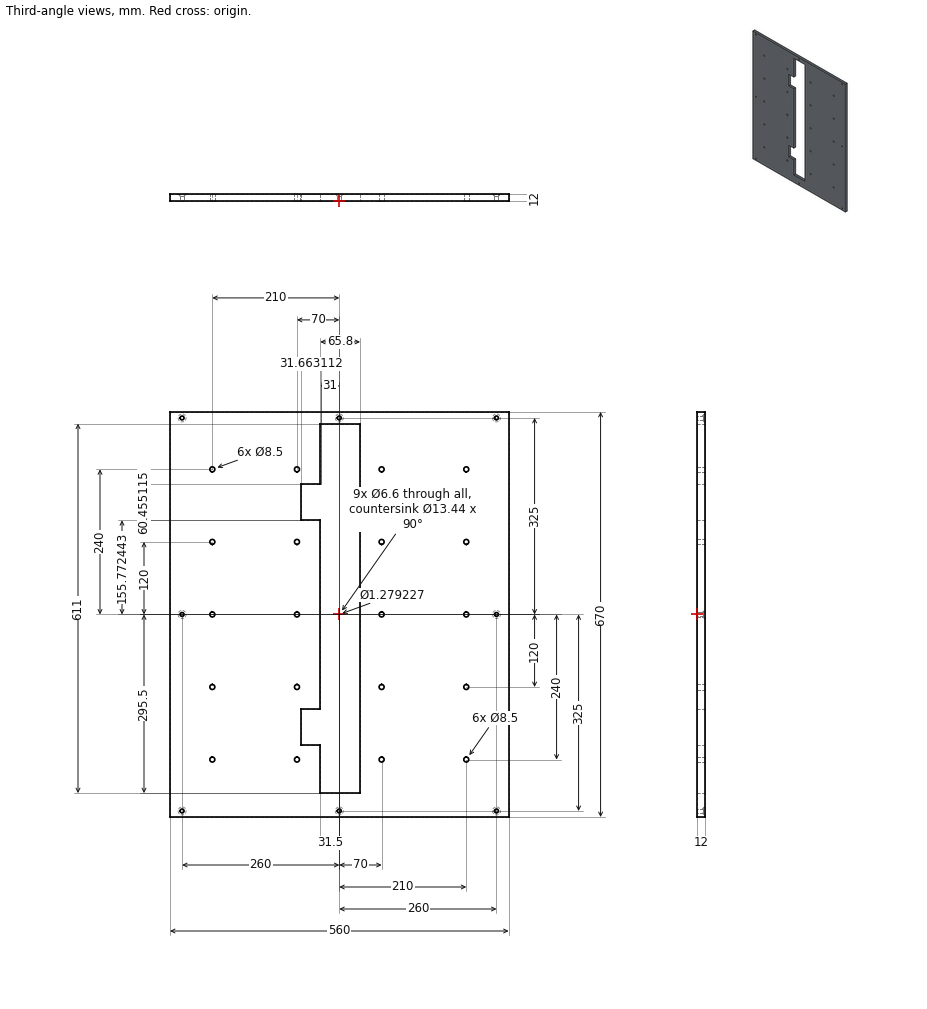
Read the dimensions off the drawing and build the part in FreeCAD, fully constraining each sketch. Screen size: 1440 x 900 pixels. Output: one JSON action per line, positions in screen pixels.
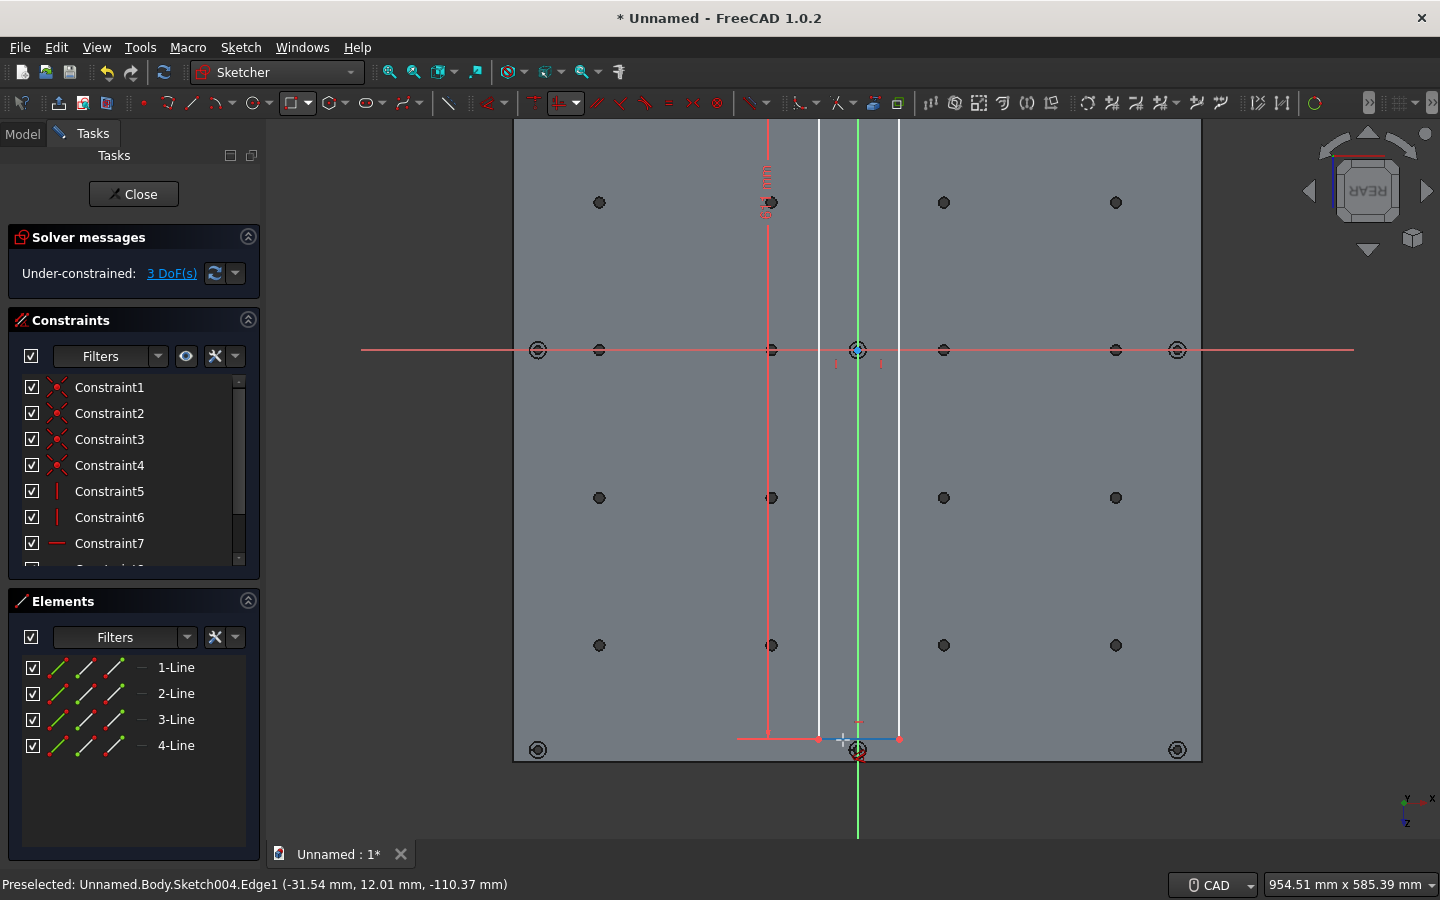
{"action": "left_click", "coordinate": [843, 739]}
{"action": "left_click", "coordinate": [841, 773]}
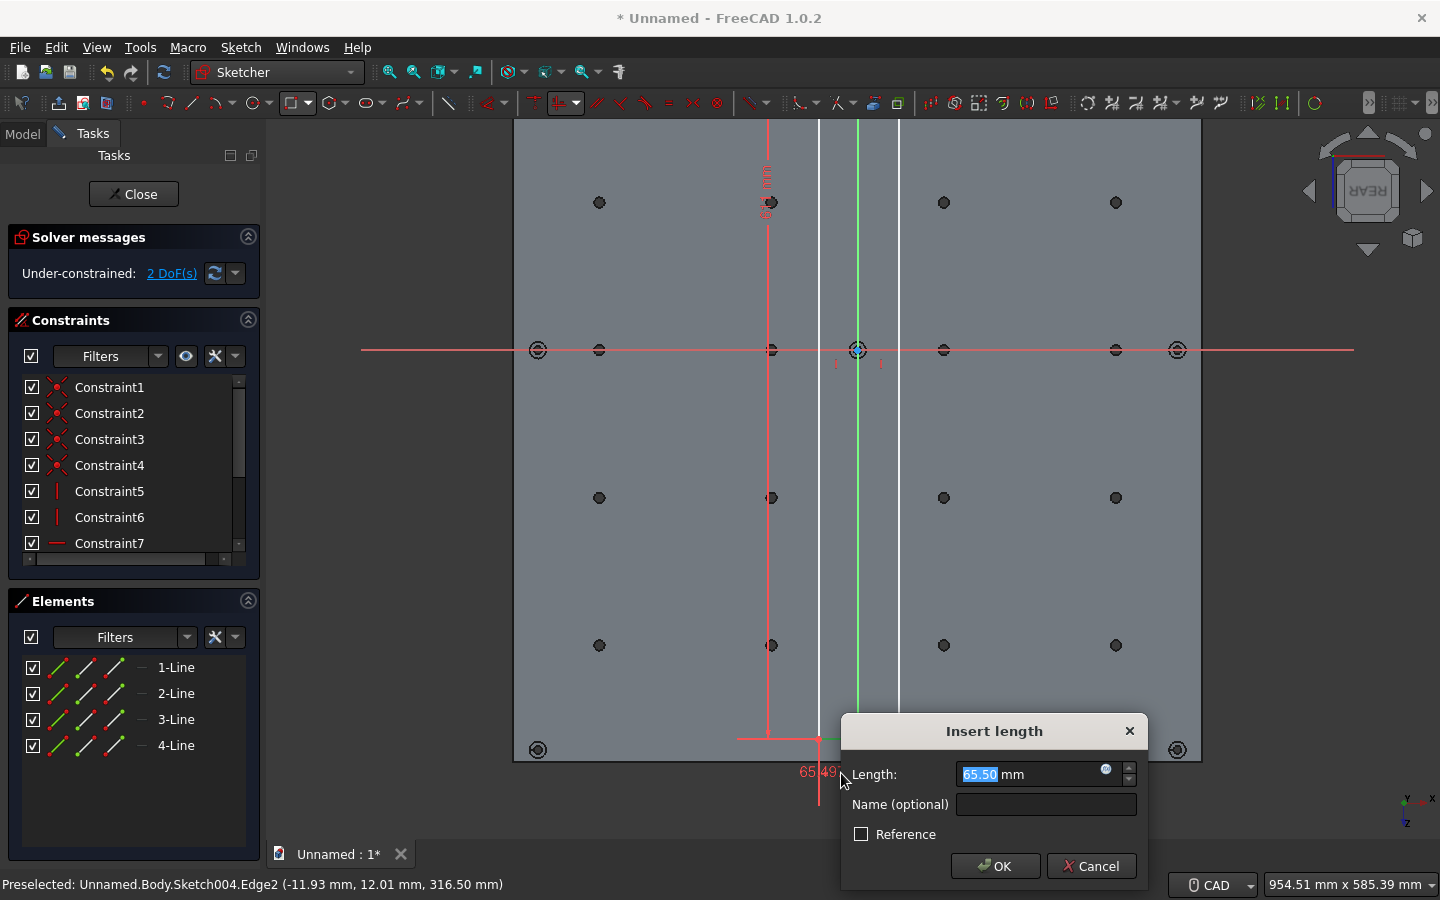
{"action": "type", "text": "65.8"}
{"action": "key", "text": "Return"}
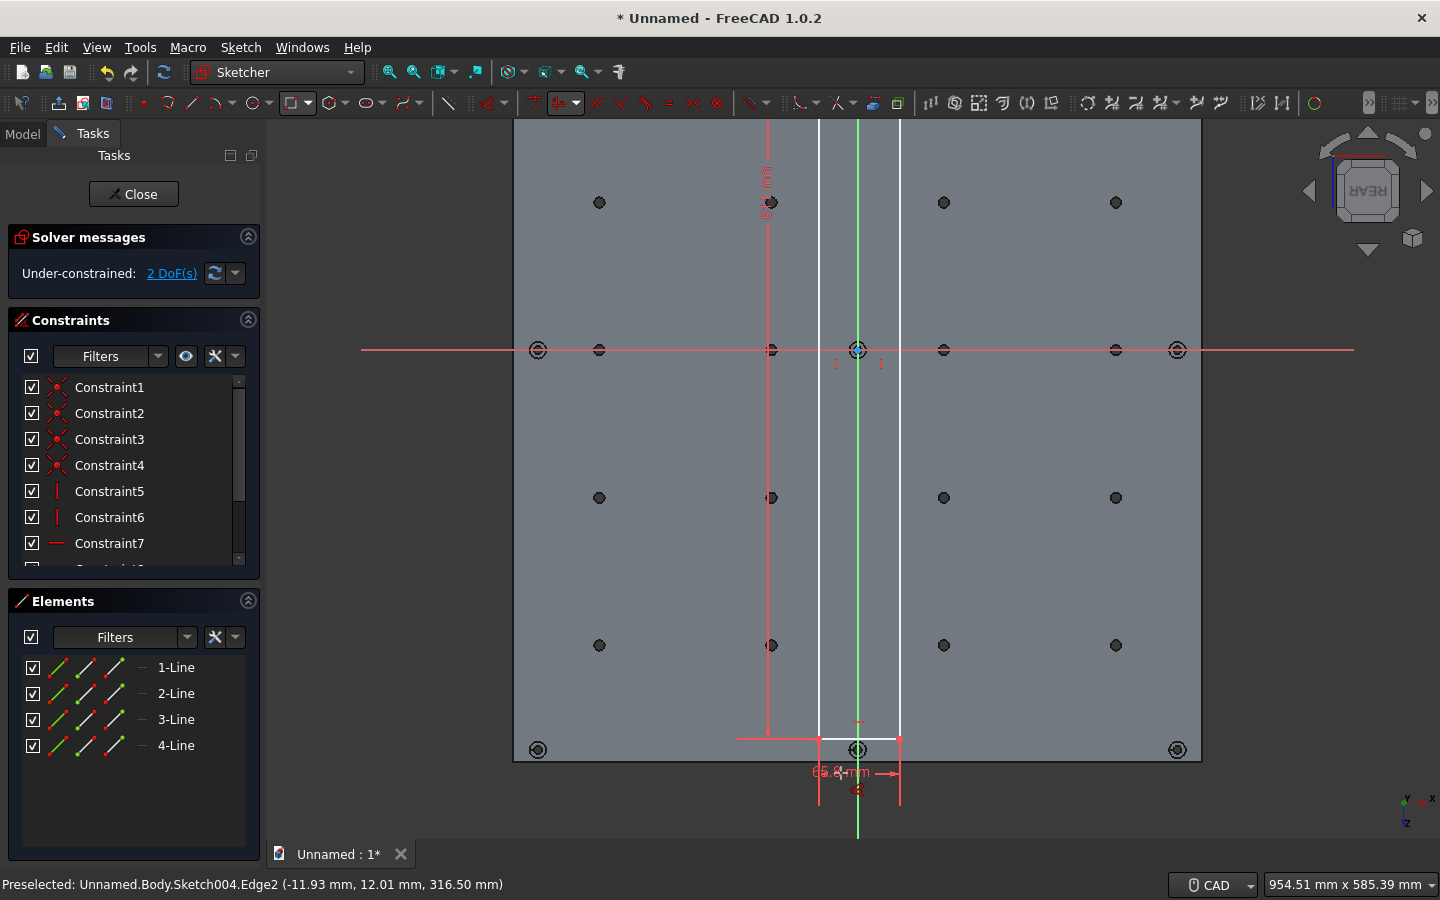
{"action": "scroll", "coordinate": [632, 716], "scroll_direction": "down", "scroll_amount": 2}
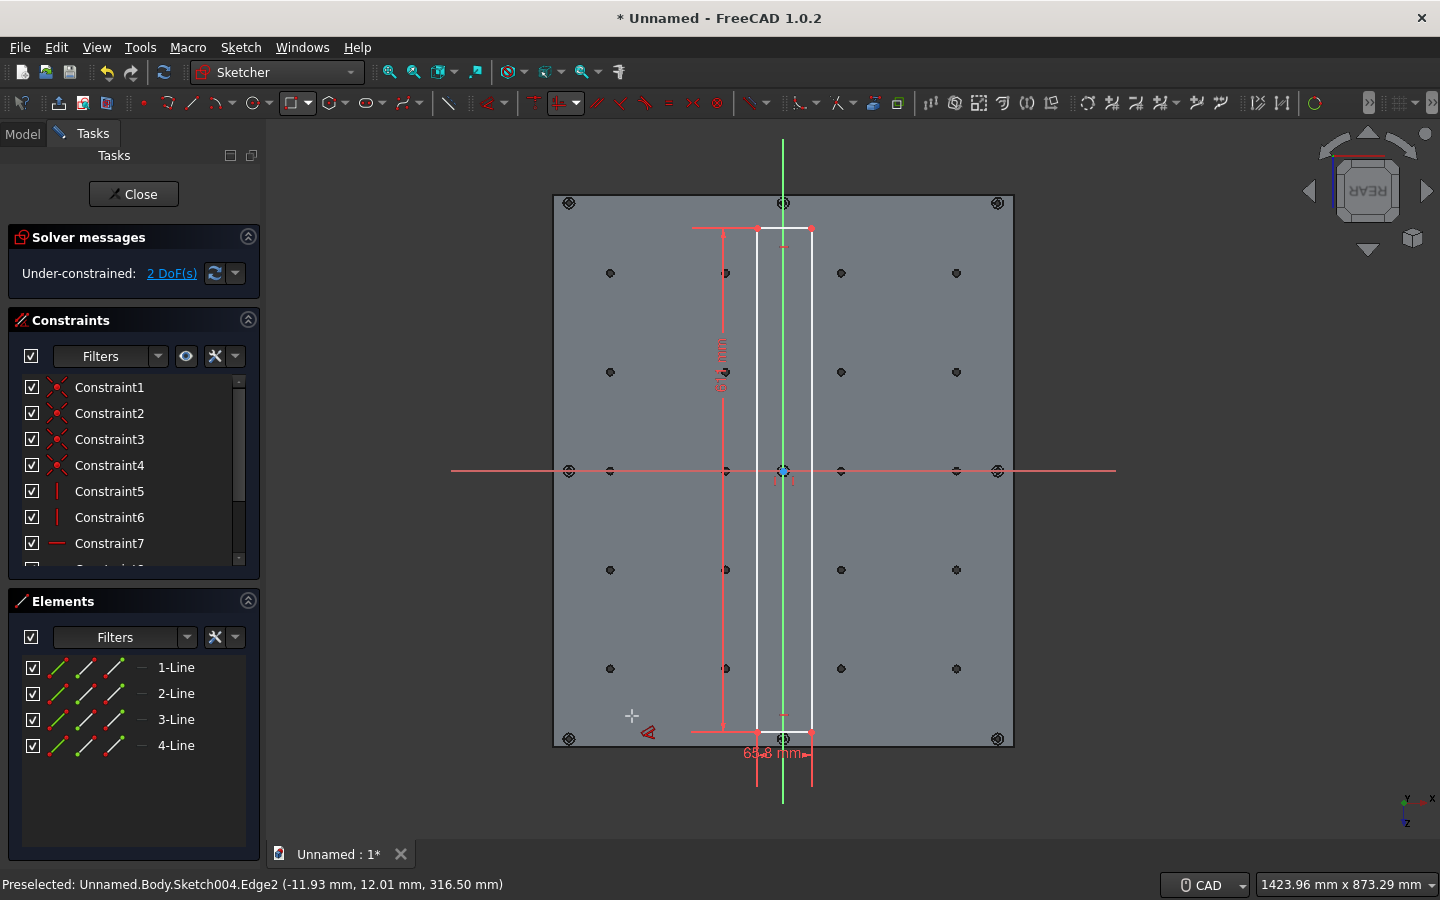
{"action": "scroll", "coordinate": [757, 228], "scroll_direction": "up", "scroll_amount": 3}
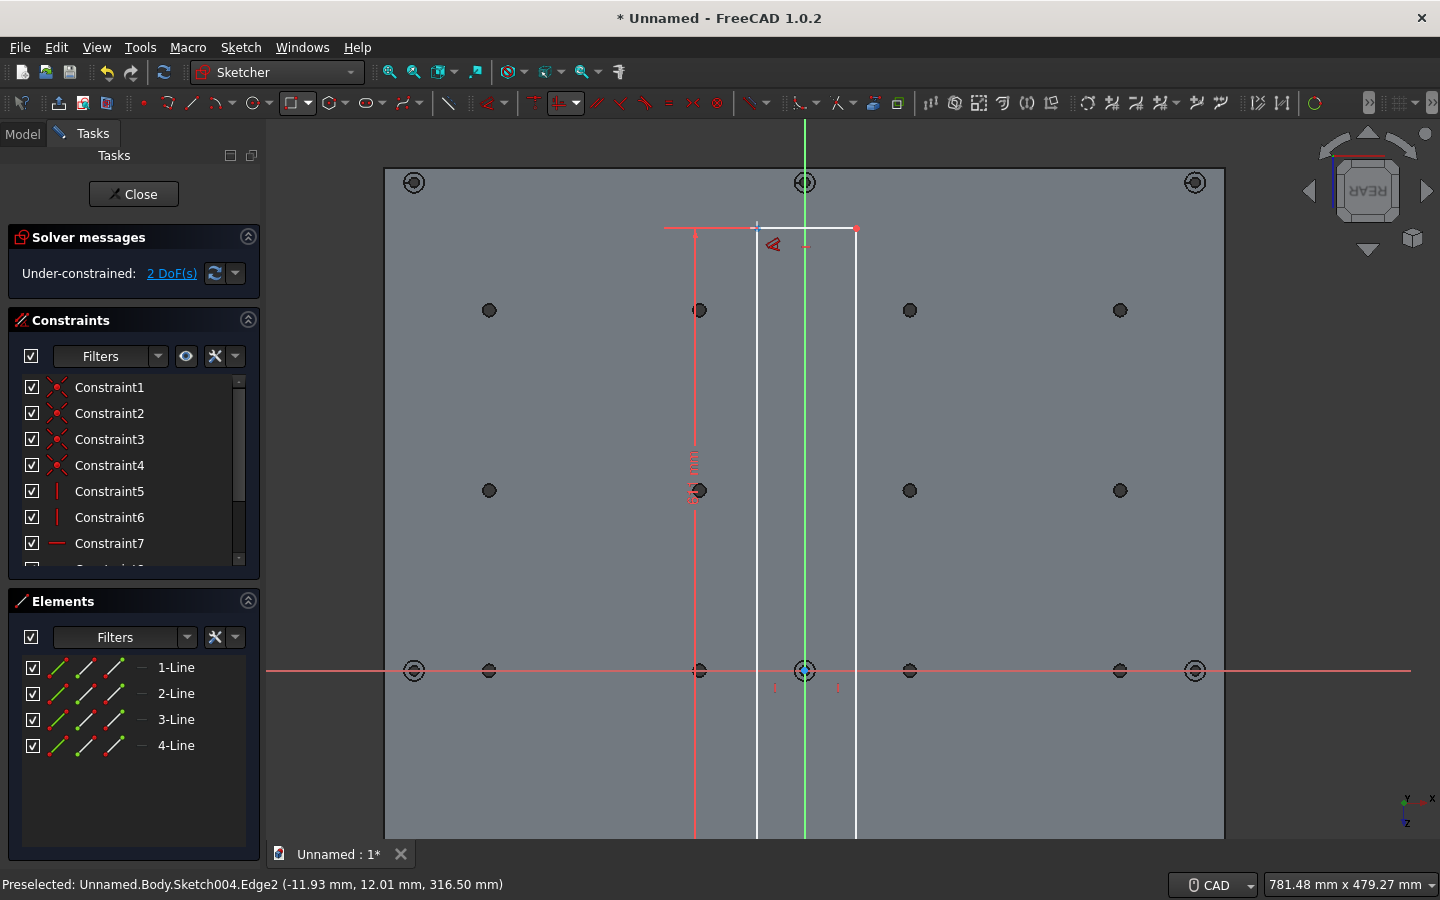
{"action": "left_click", "coordinate": [757, 228]}
{"action": "left_click", "coordinate": [781, 194]}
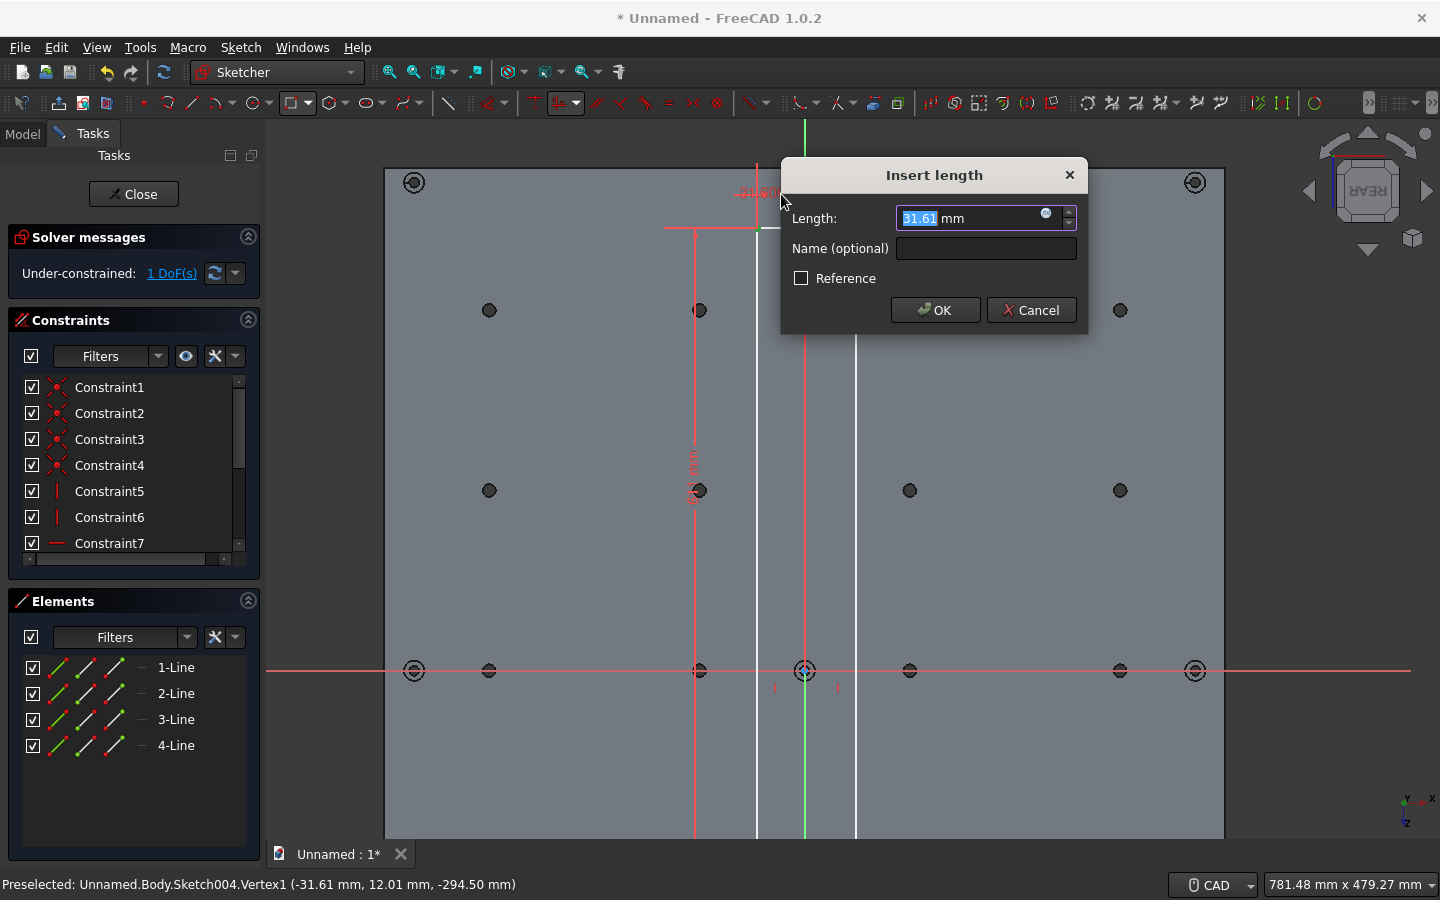
{"action": "type", "text": "31.5"}
{"action": "key", "text": "Return"}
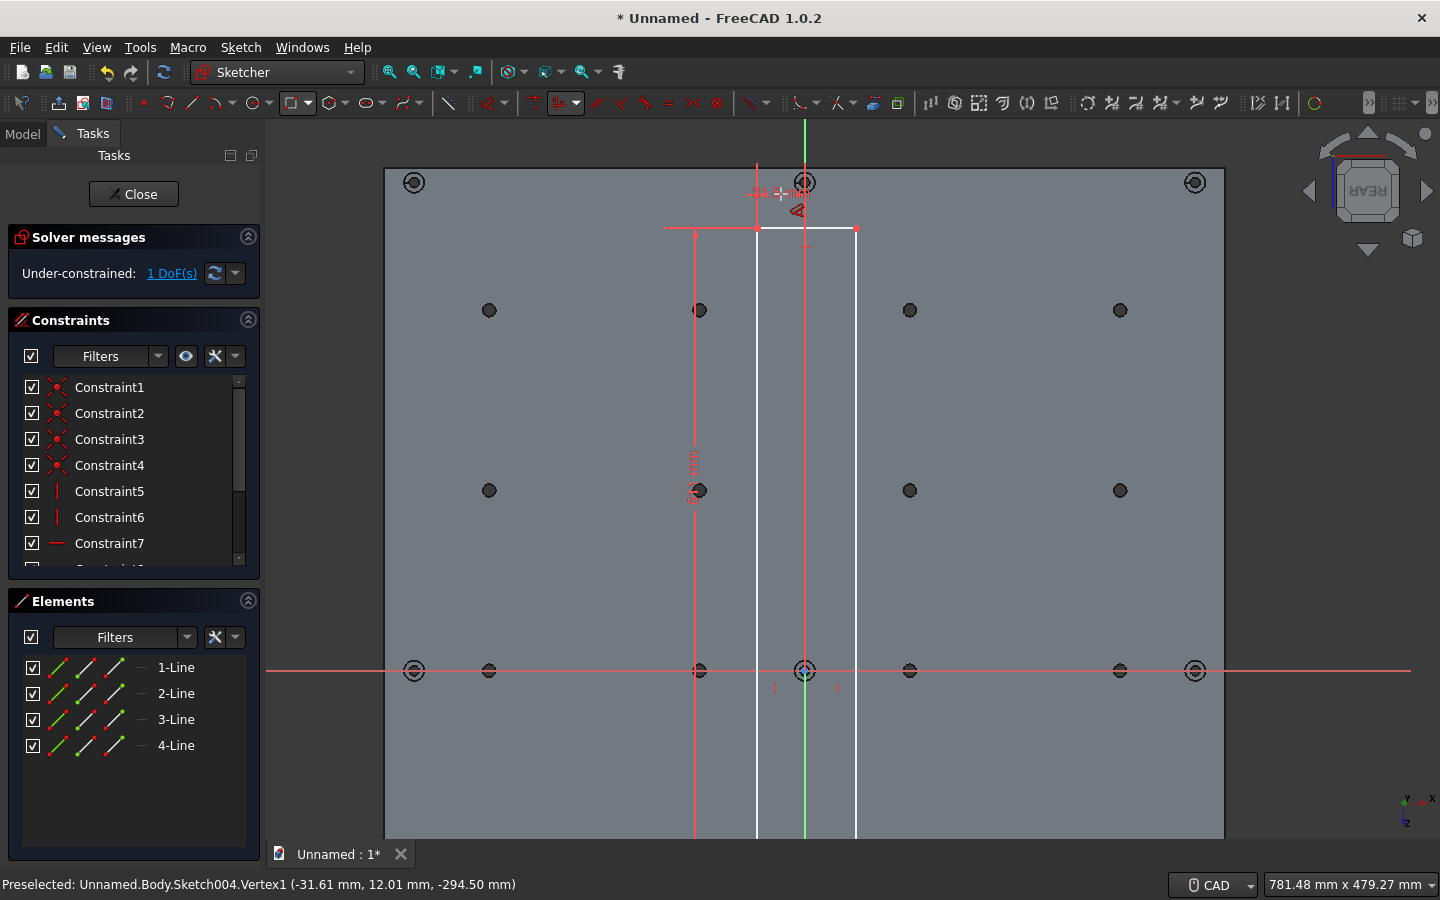
{"action": "left_click", "coordinate": [757, 228]}
{"action": "left_click", "coordinate": [723, 450]}